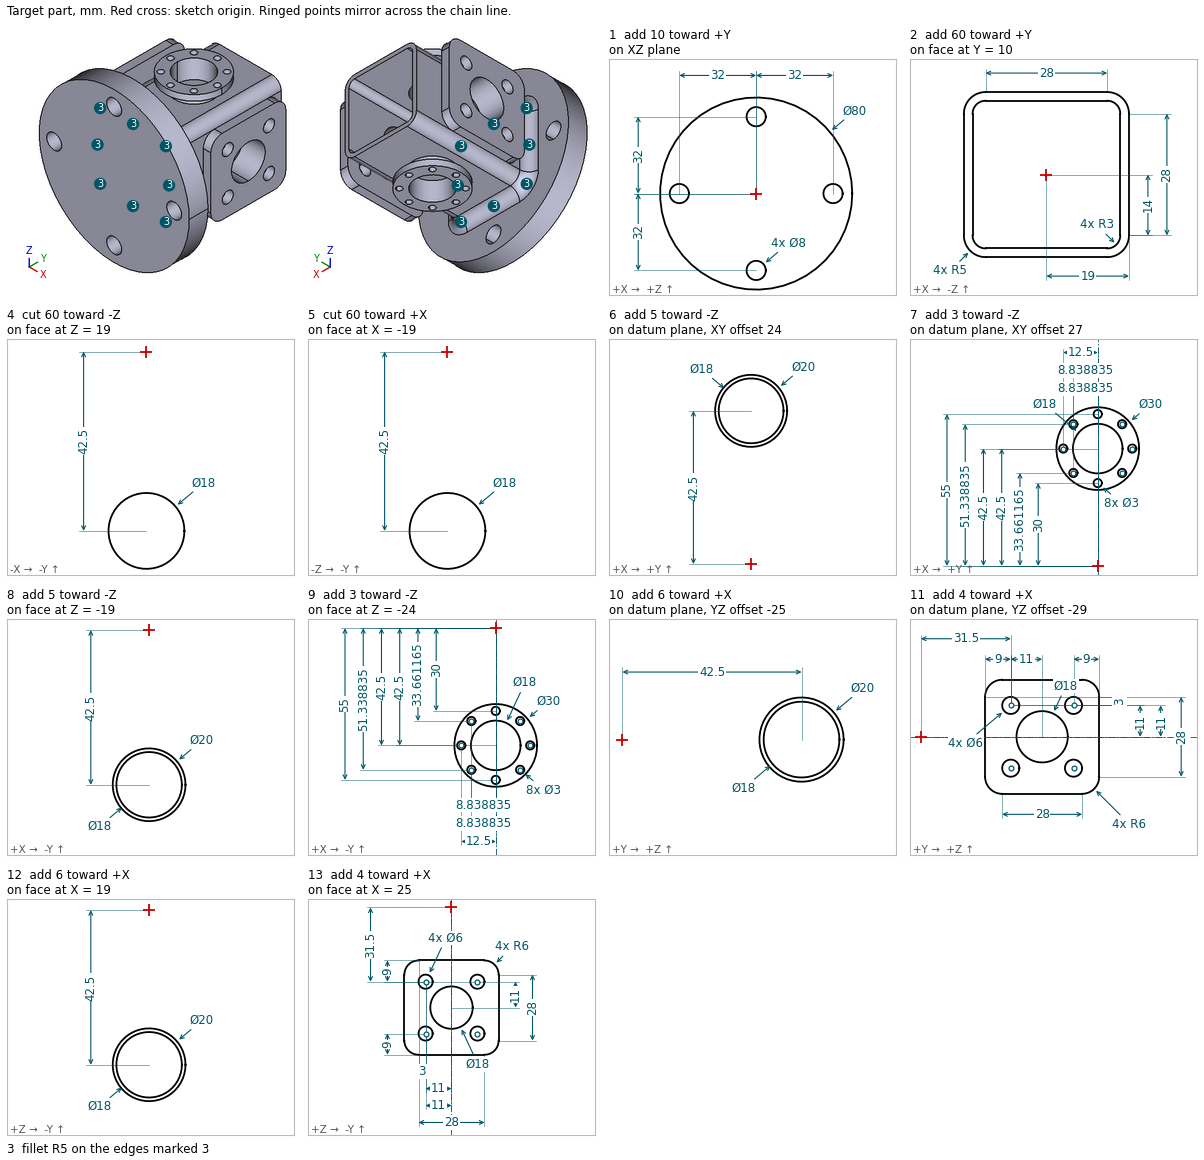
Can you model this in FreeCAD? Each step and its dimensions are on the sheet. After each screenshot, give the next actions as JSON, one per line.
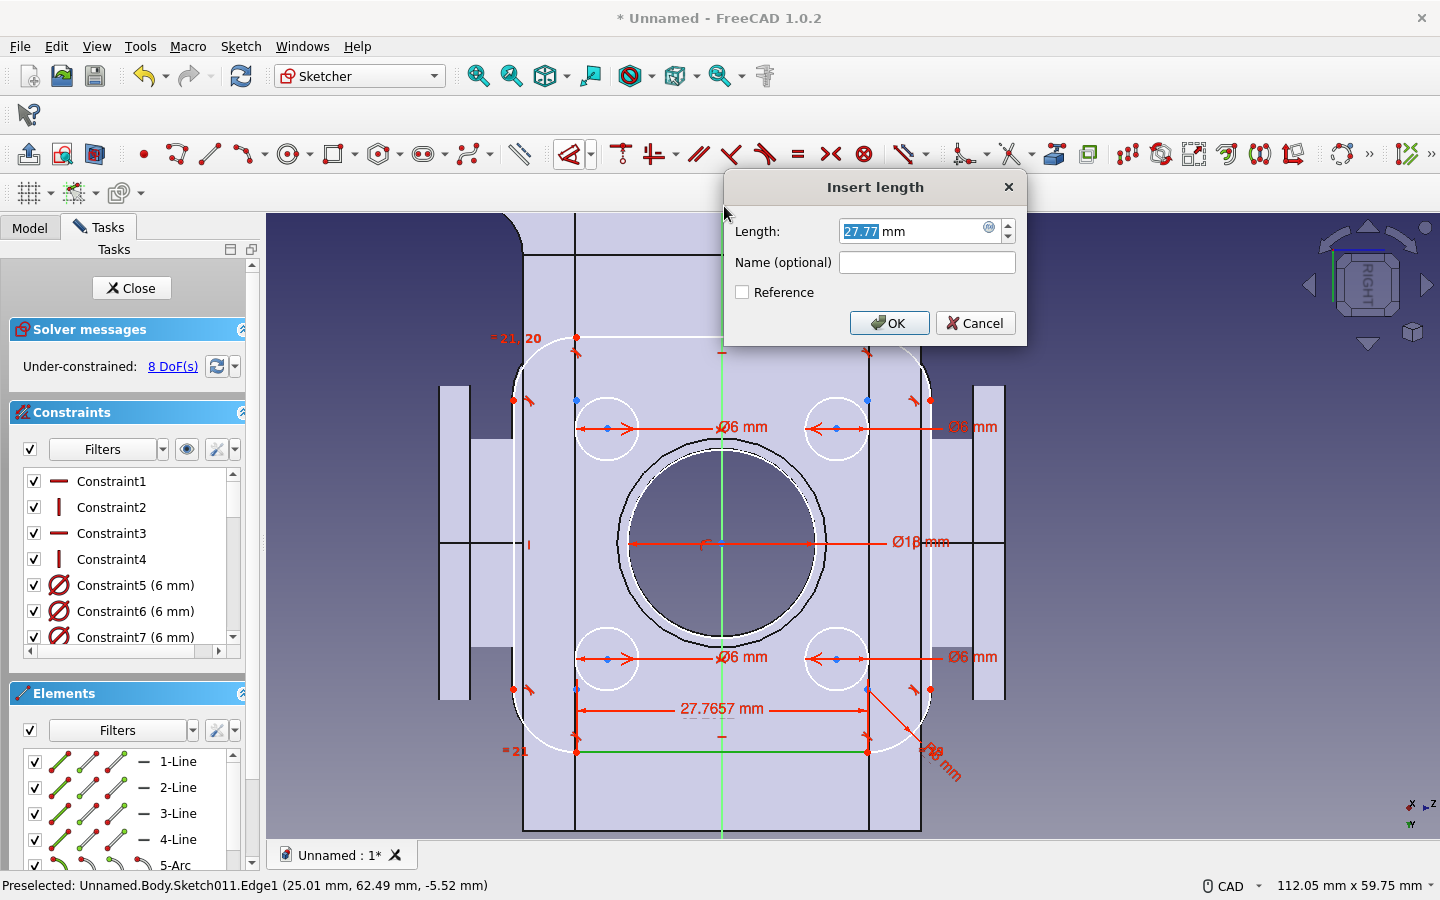
{"action": "type", "text": "28"}
{"action": "key", "text": "Return"}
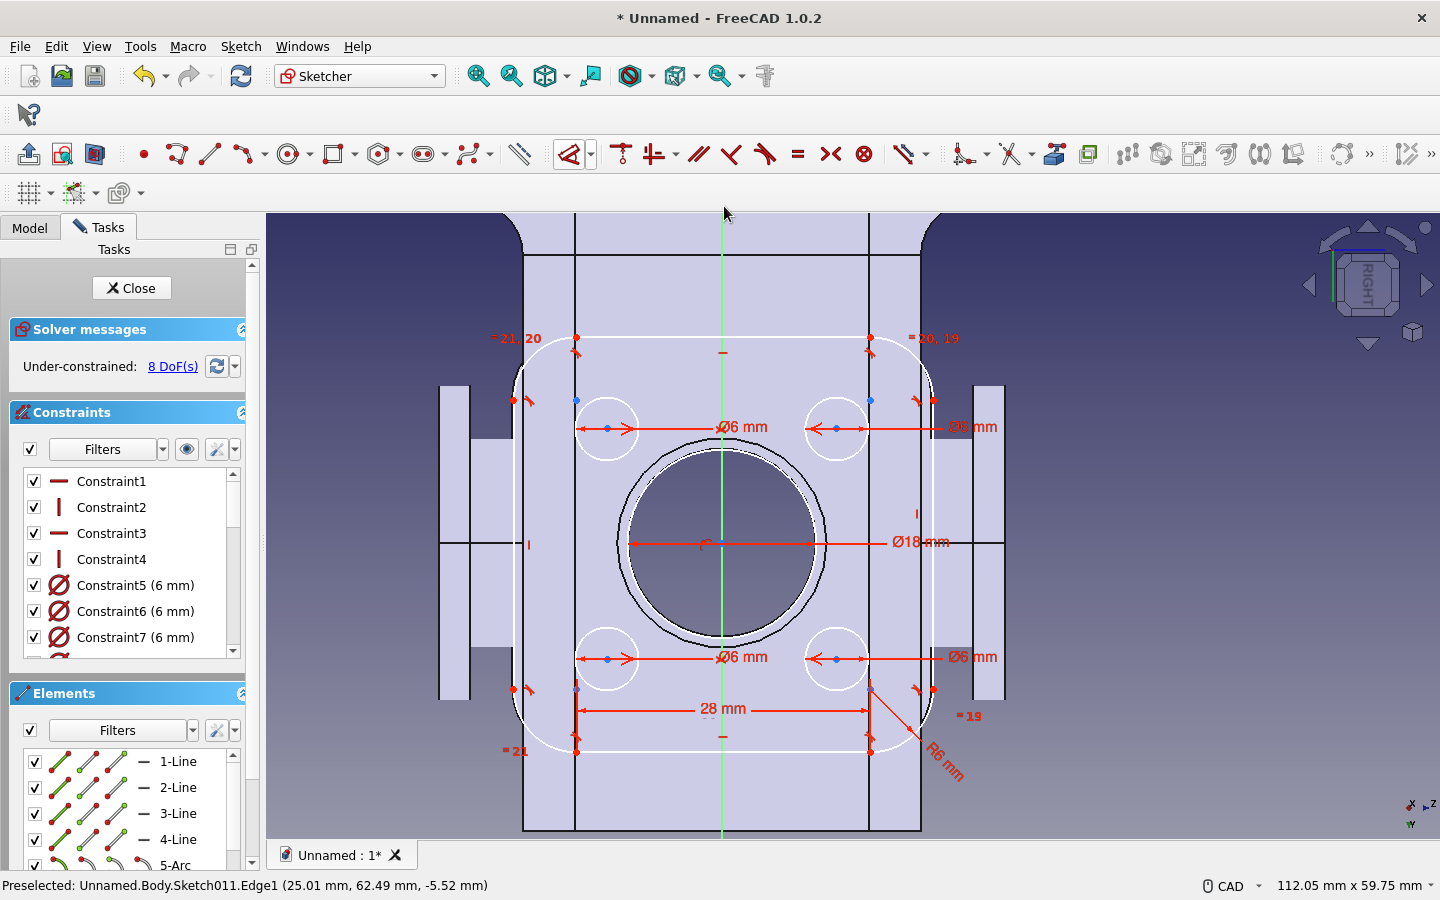
{"action": "left_click", "coordinate": [933, 603]}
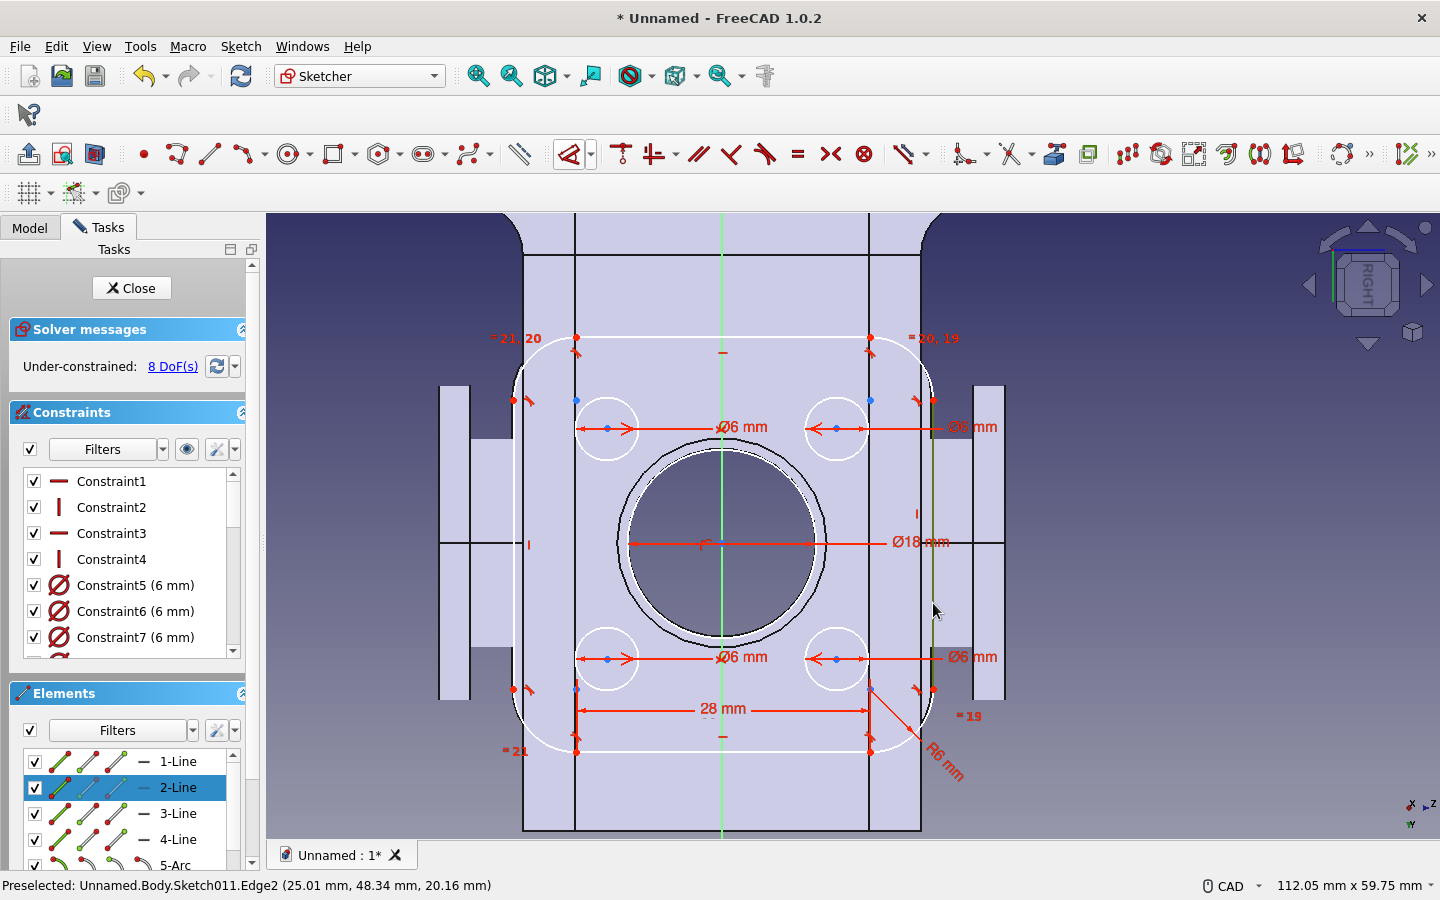
{"action": "left_click", "coordinate": [590, 154]}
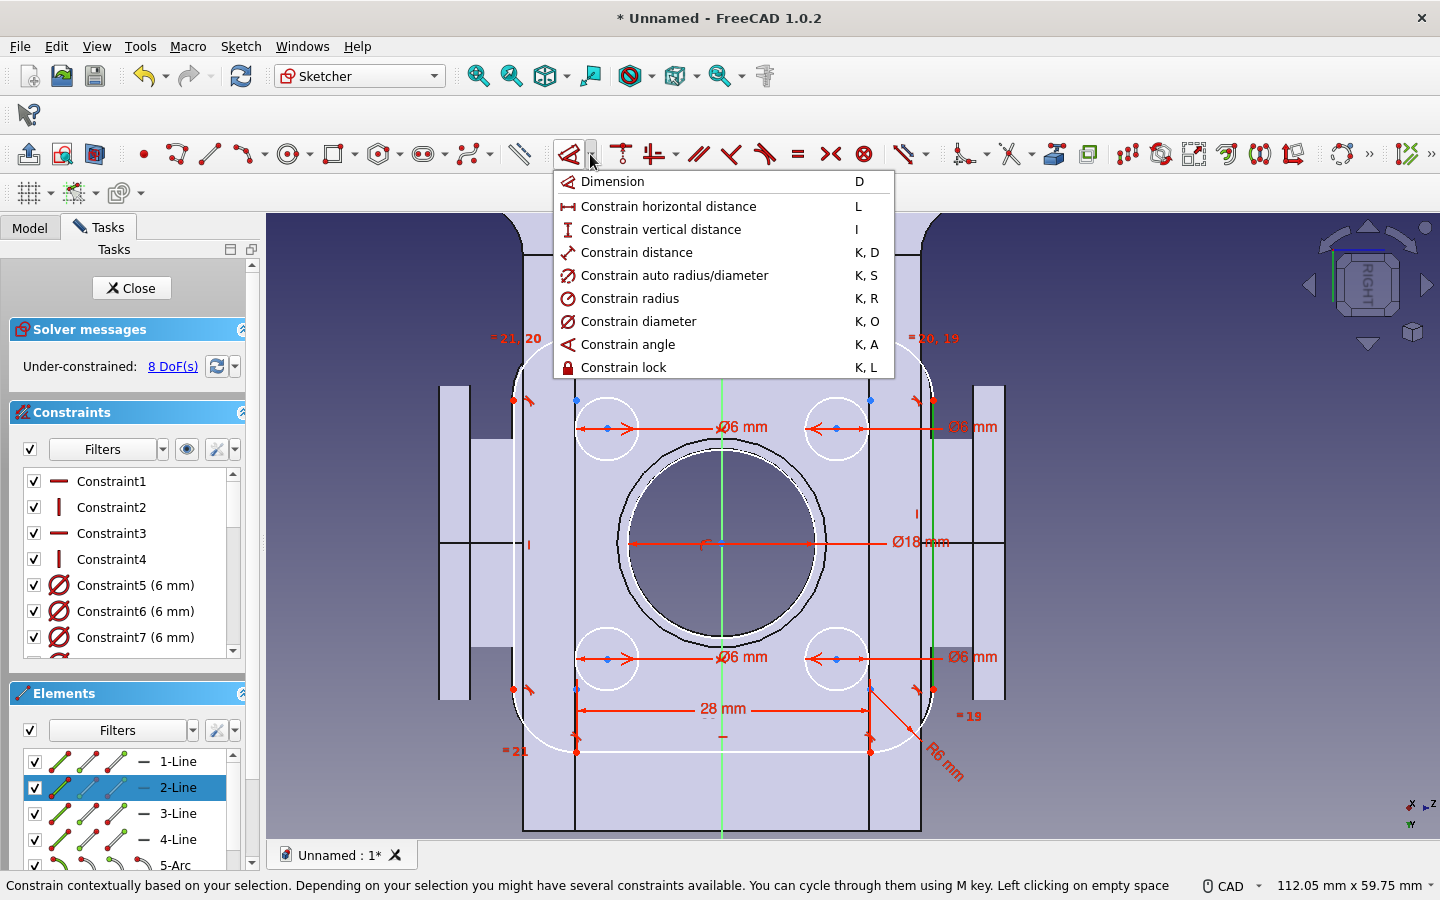
{"action": "left_click", "coordinate": [724, 230]}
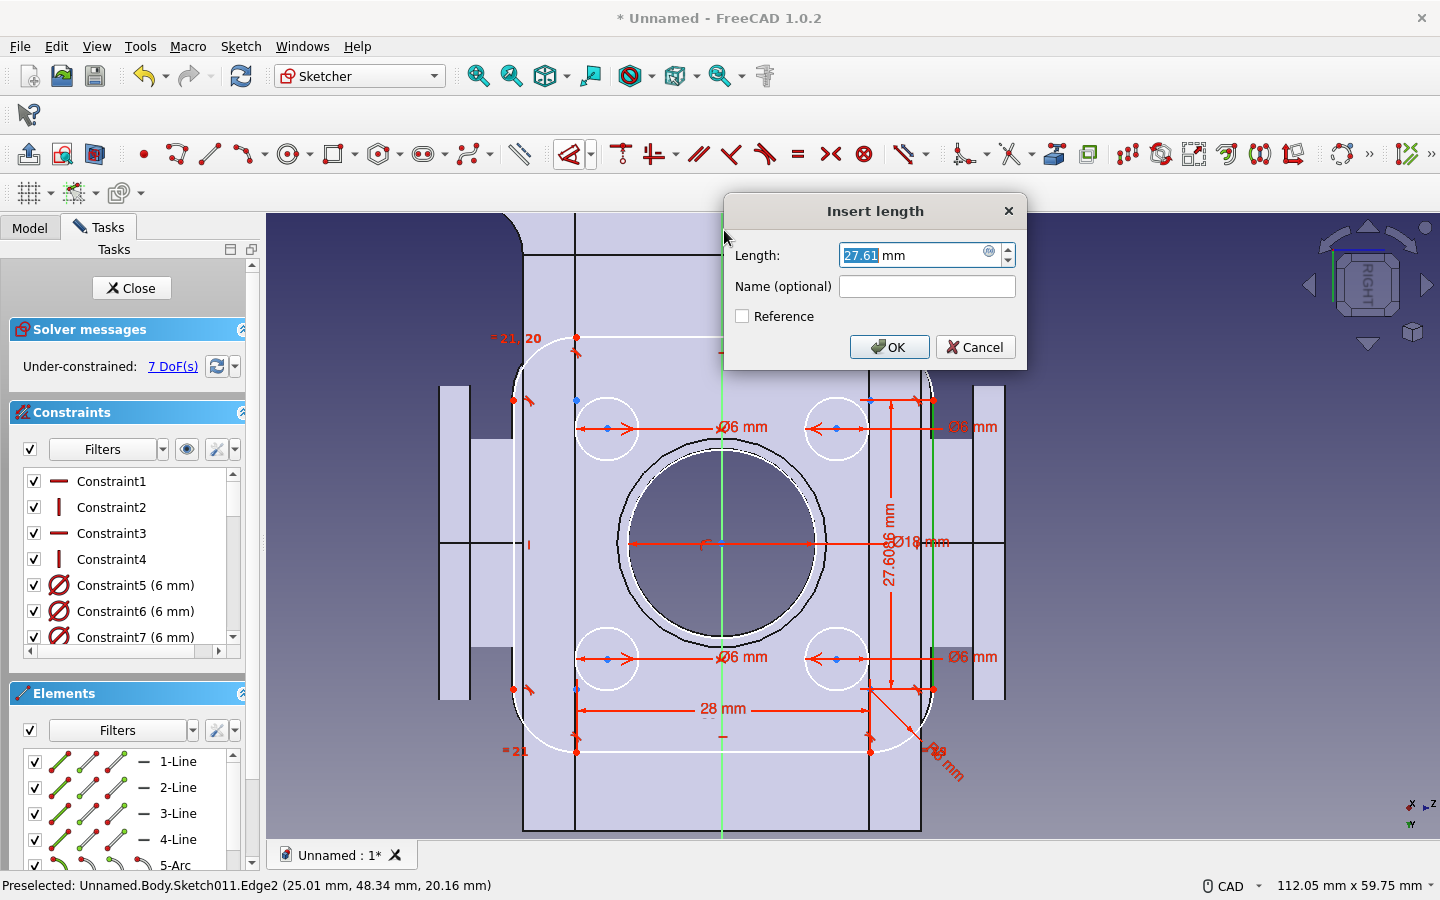
{"action": "type", "text": "28"}
{"action": "key", "text": "Return"}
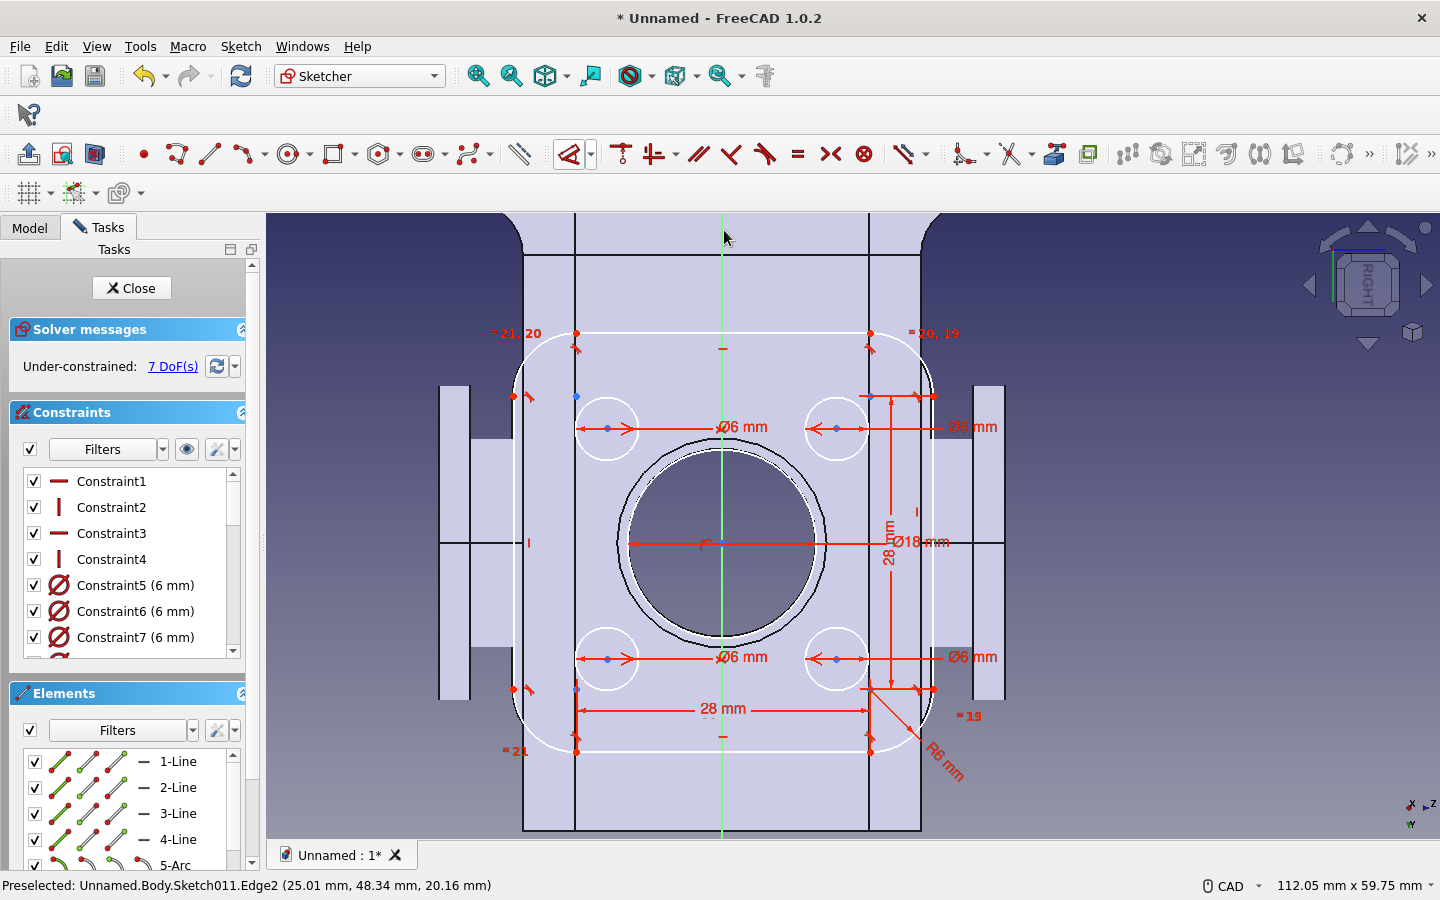
{"action": "left_click", "coordinate": [607, 429]}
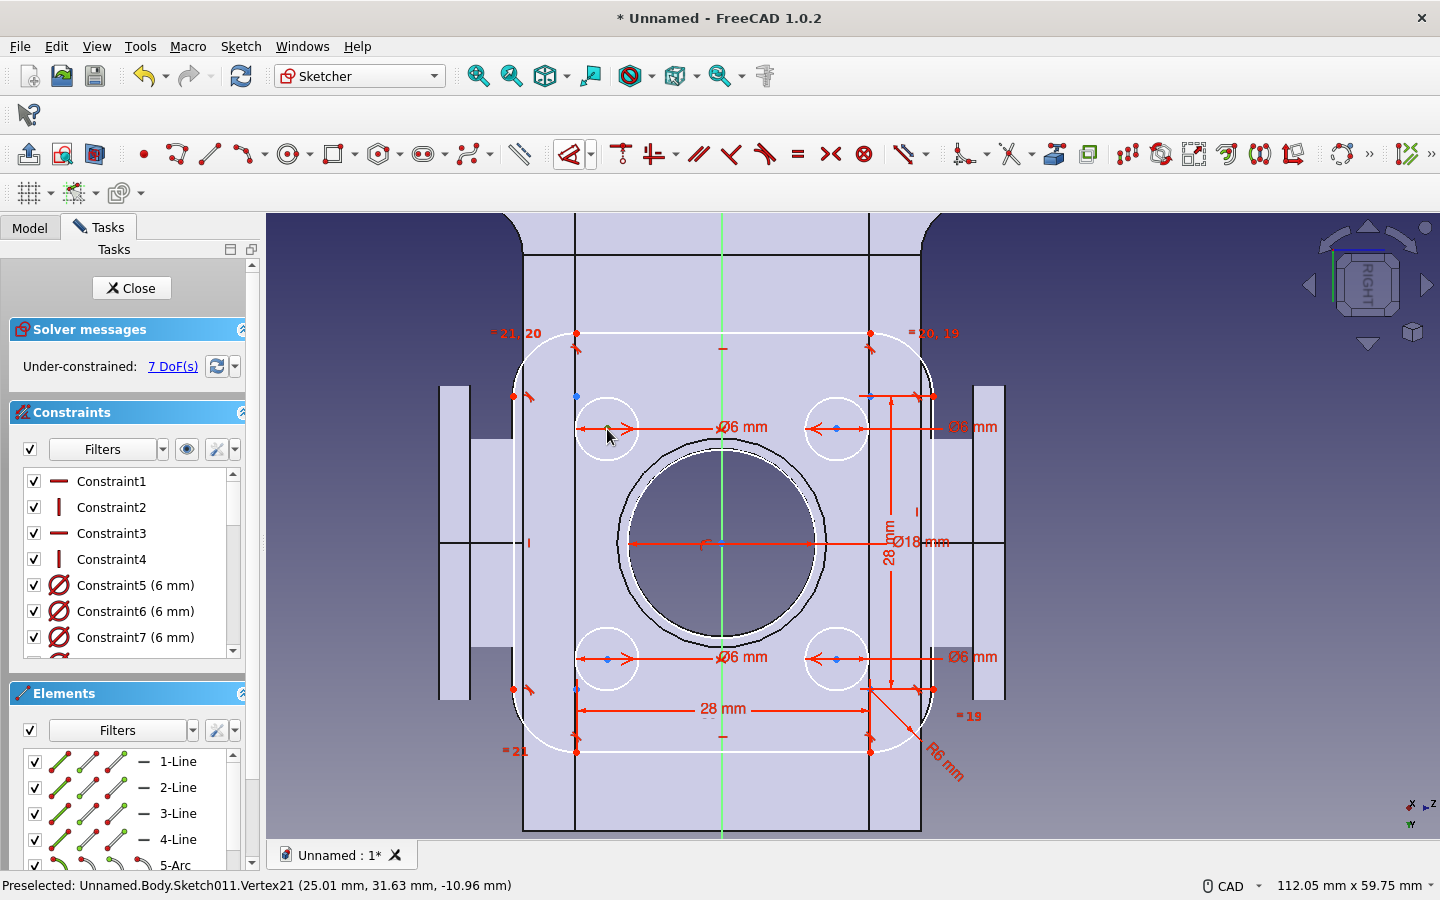
{"action": "key", "text": "l"}